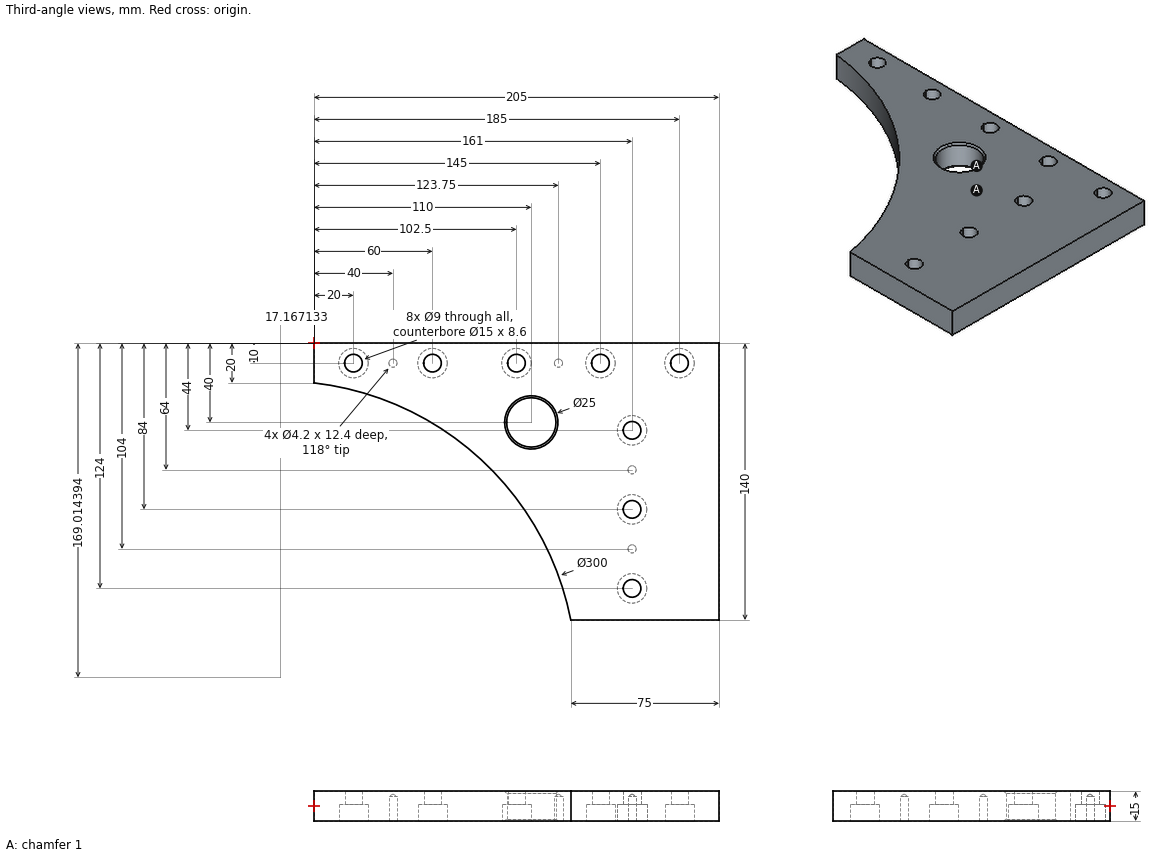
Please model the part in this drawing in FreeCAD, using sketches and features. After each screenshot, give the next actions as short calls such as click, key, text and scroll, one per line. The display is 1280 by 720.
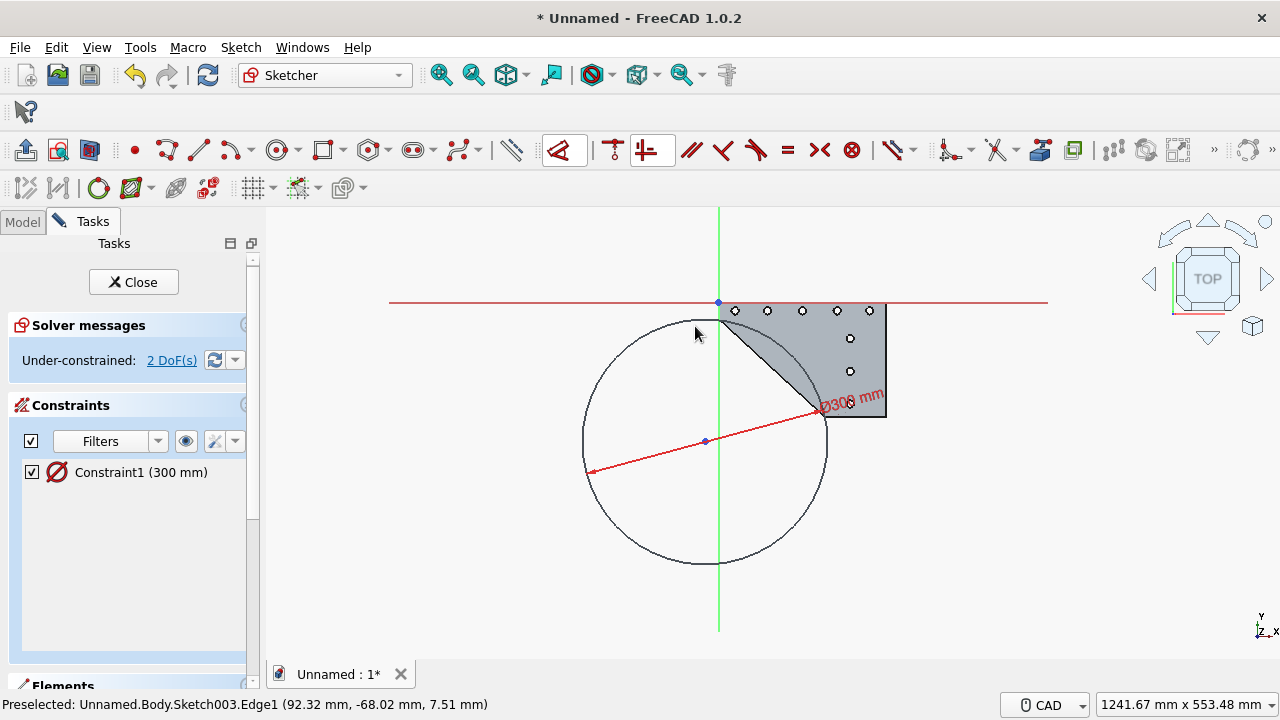
scroll(705, 442, up, 6)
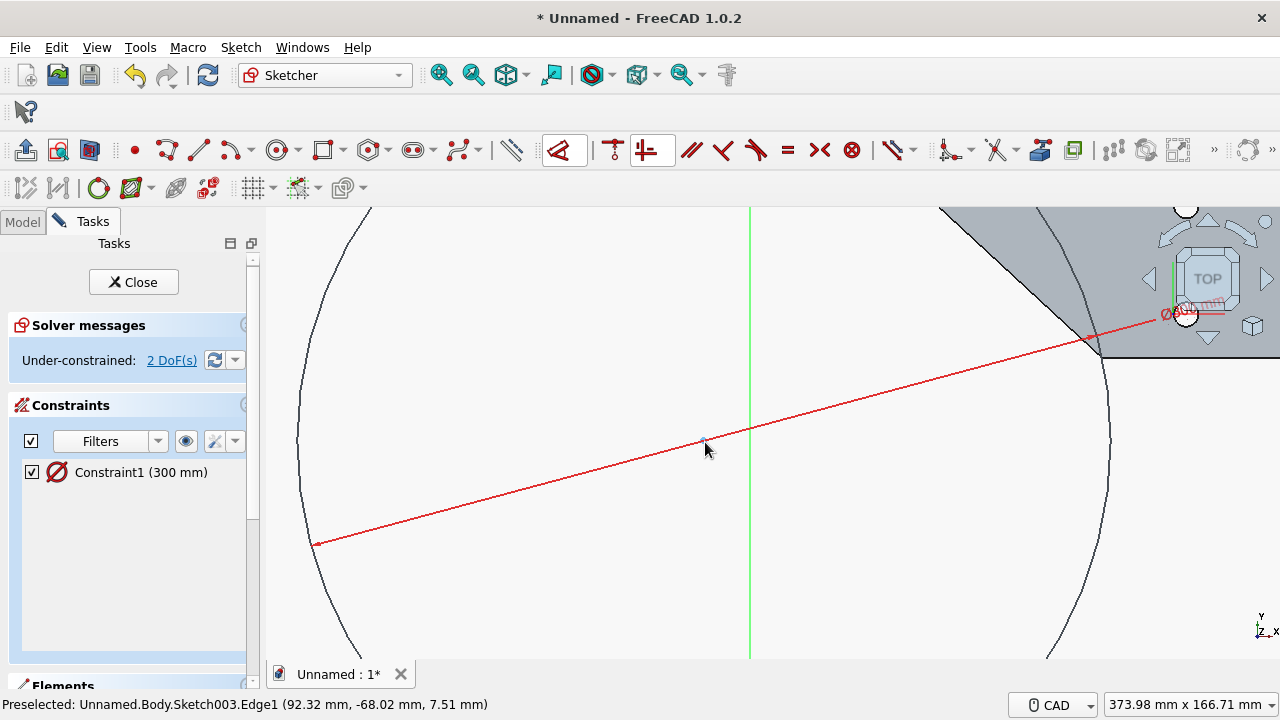
click(704, 441)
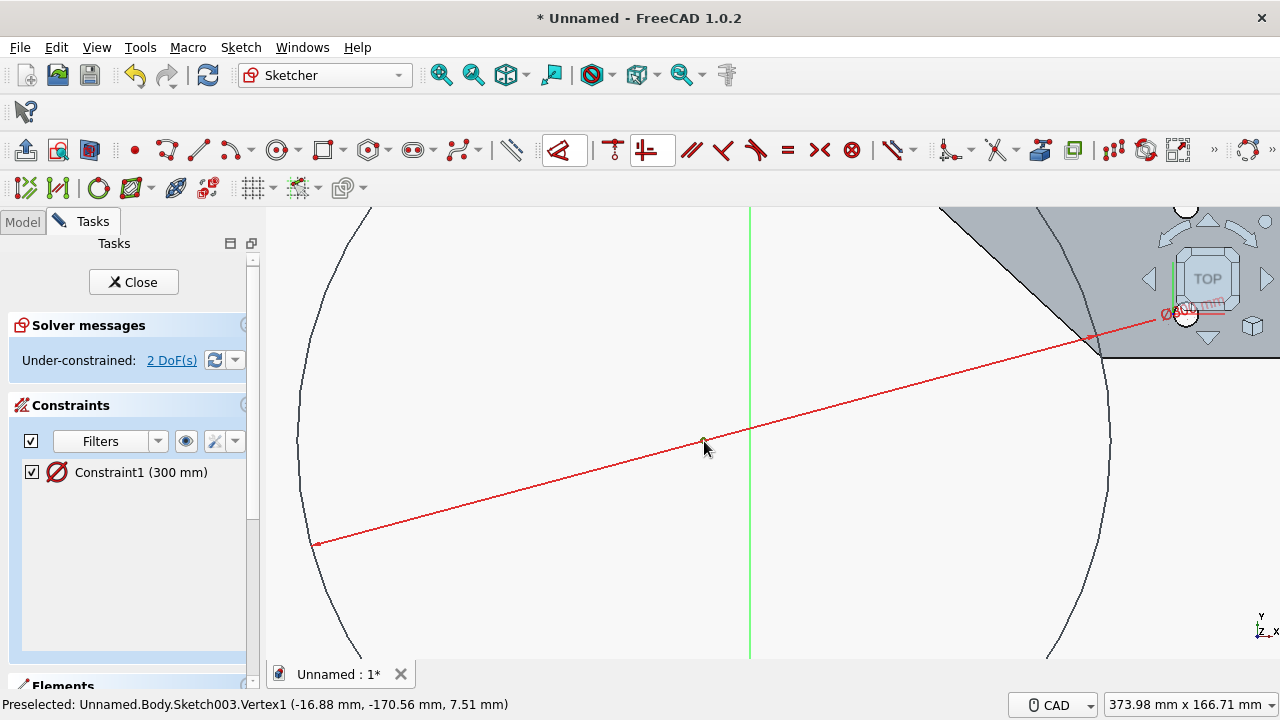
key(l)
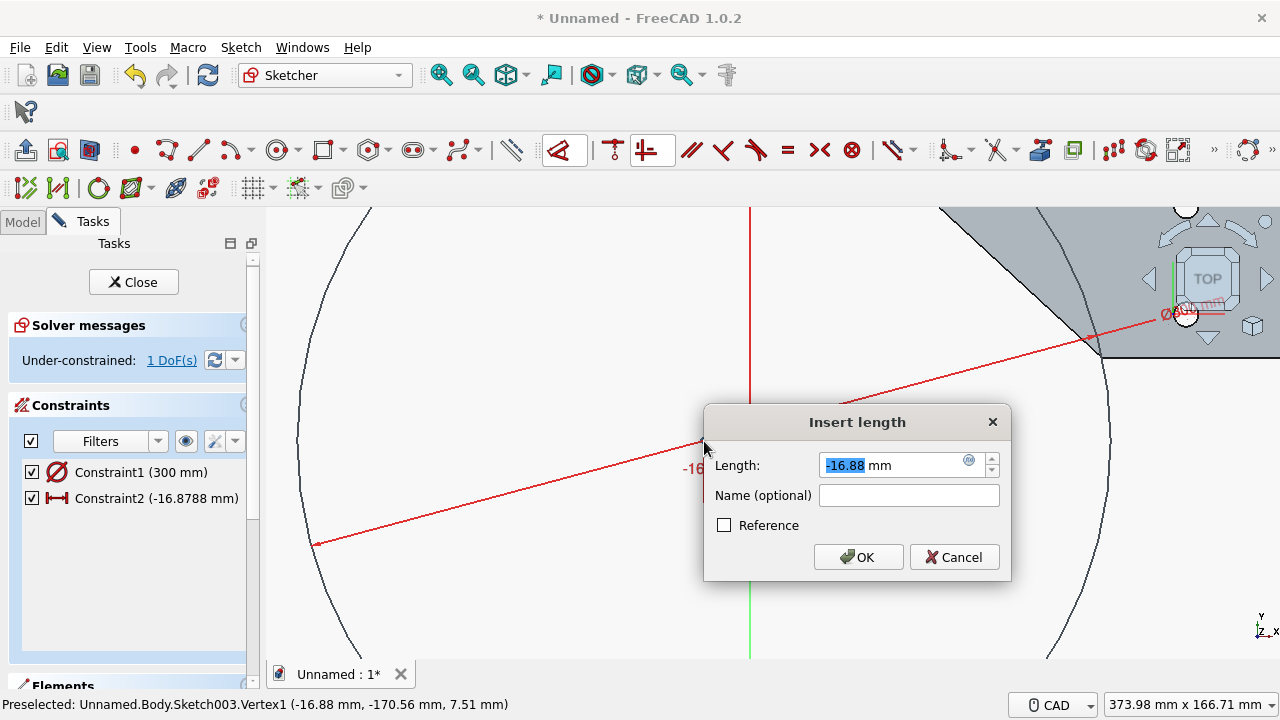
text(-17.167133)
key(Return)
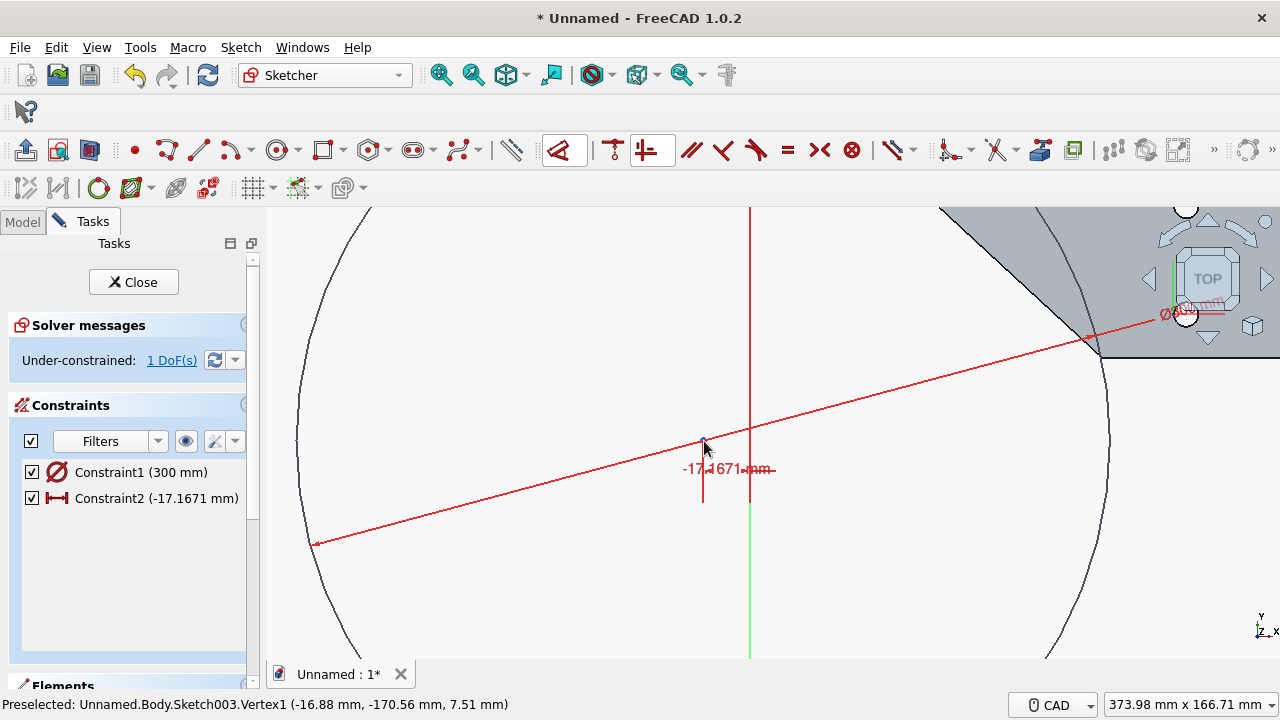
click(703, 441)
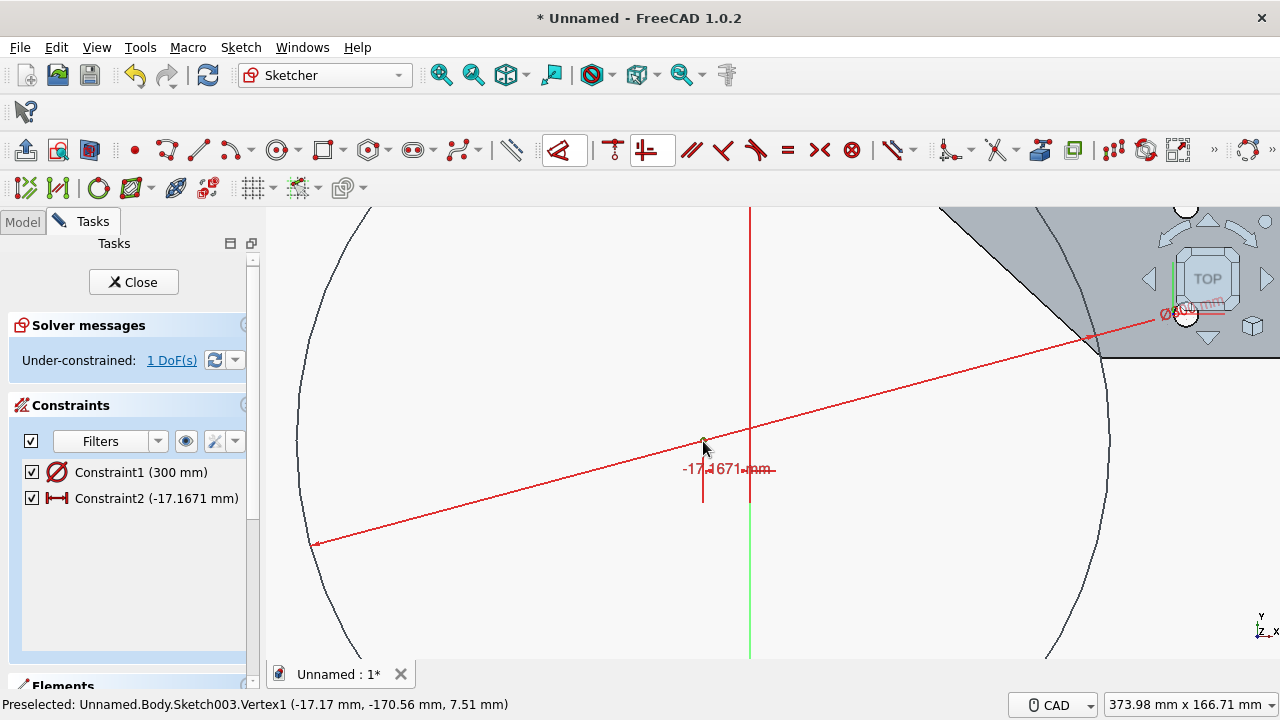
click(582, 150)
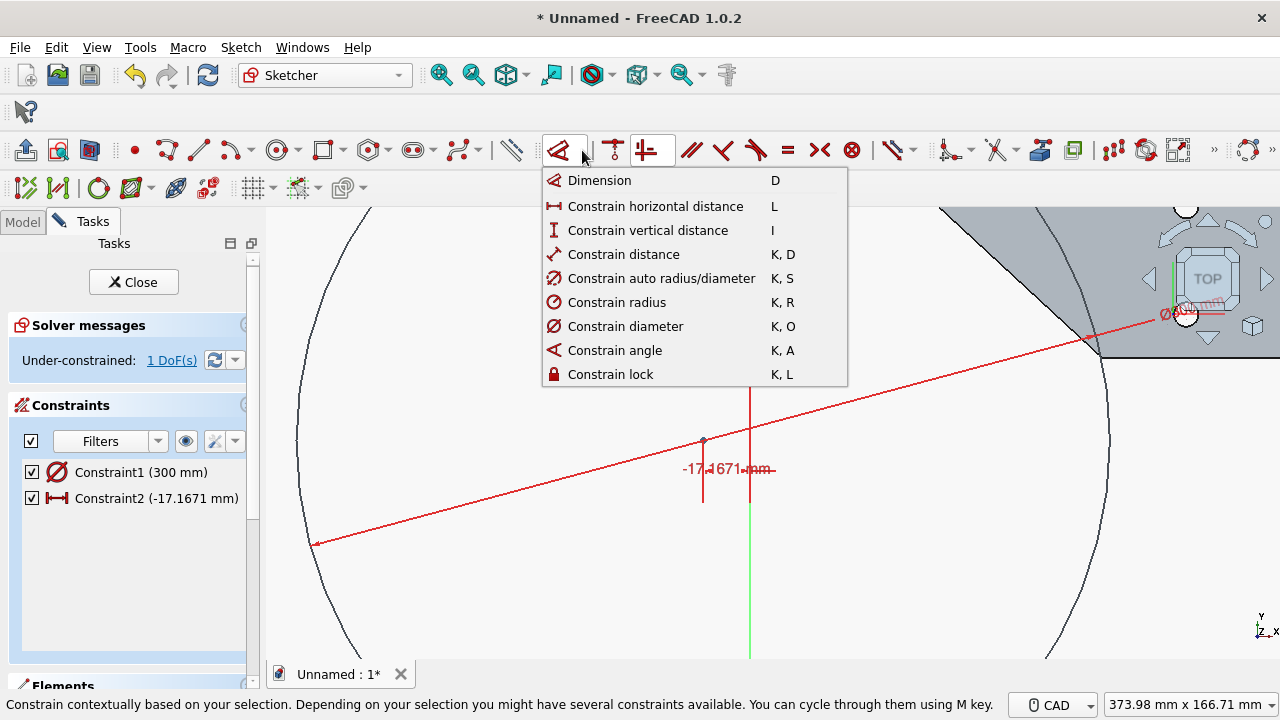
click(695, 230)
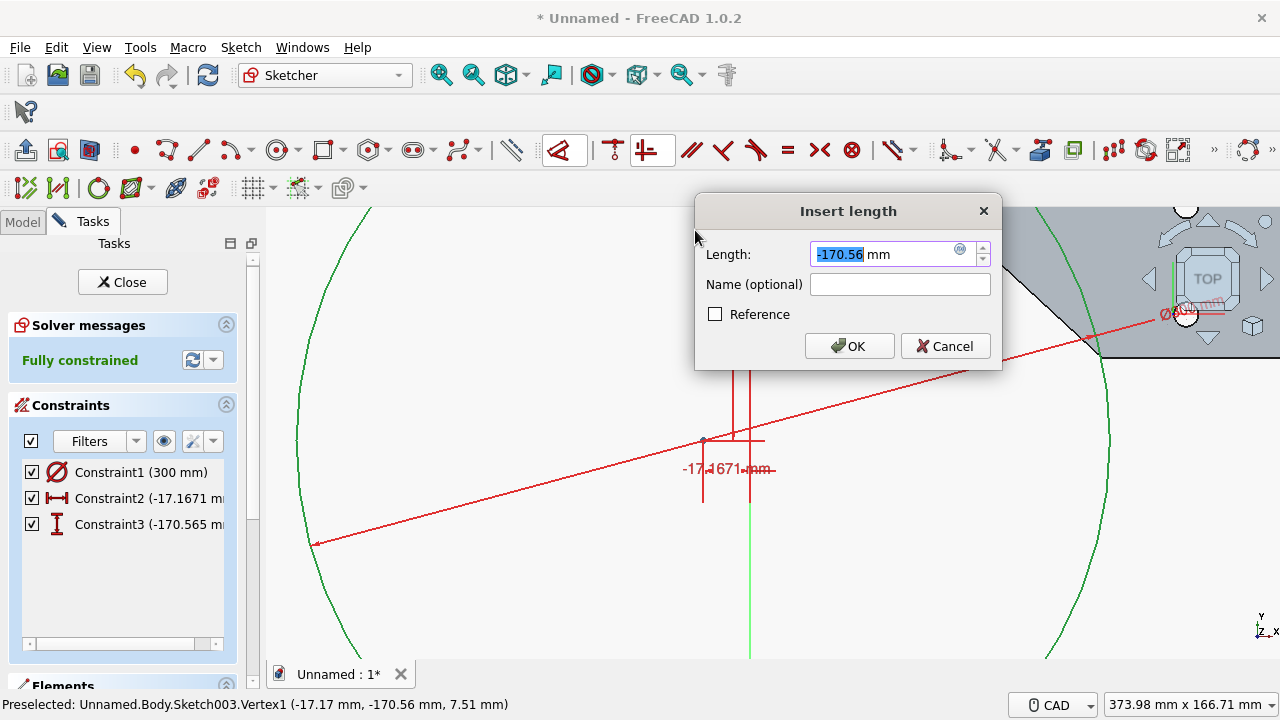
text(-169.014394)
key(Return)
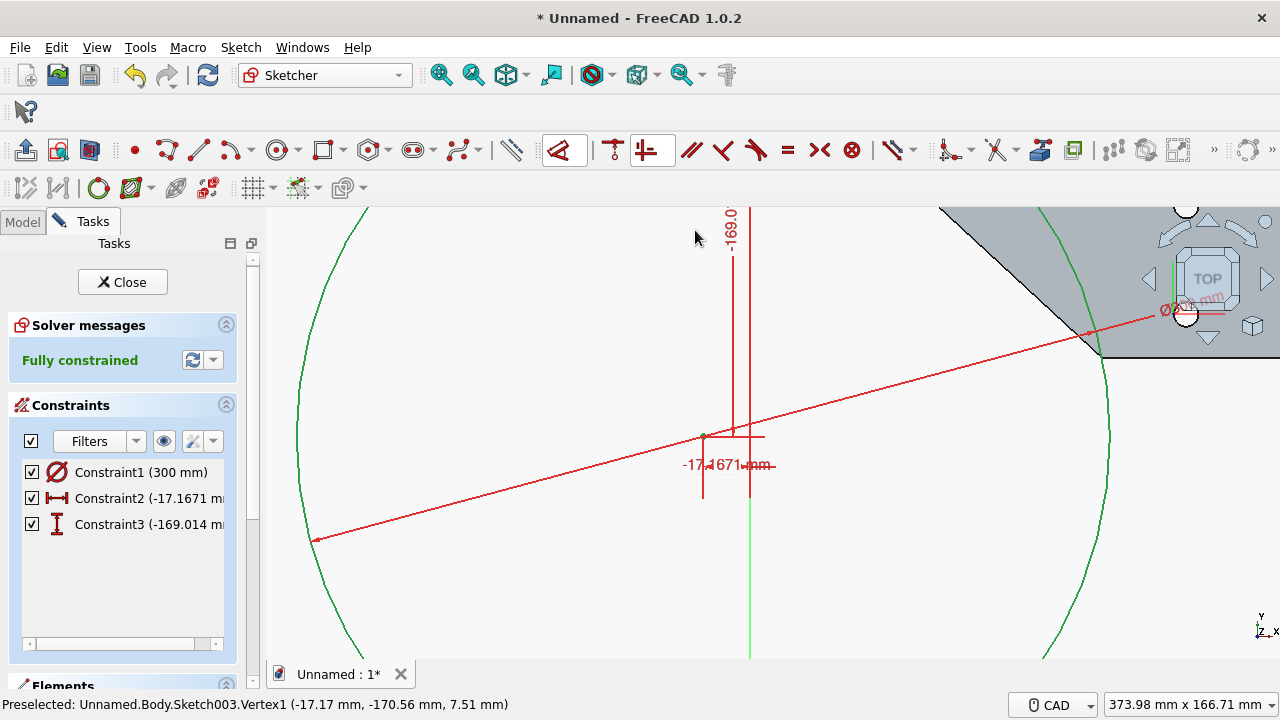
click(123, 282)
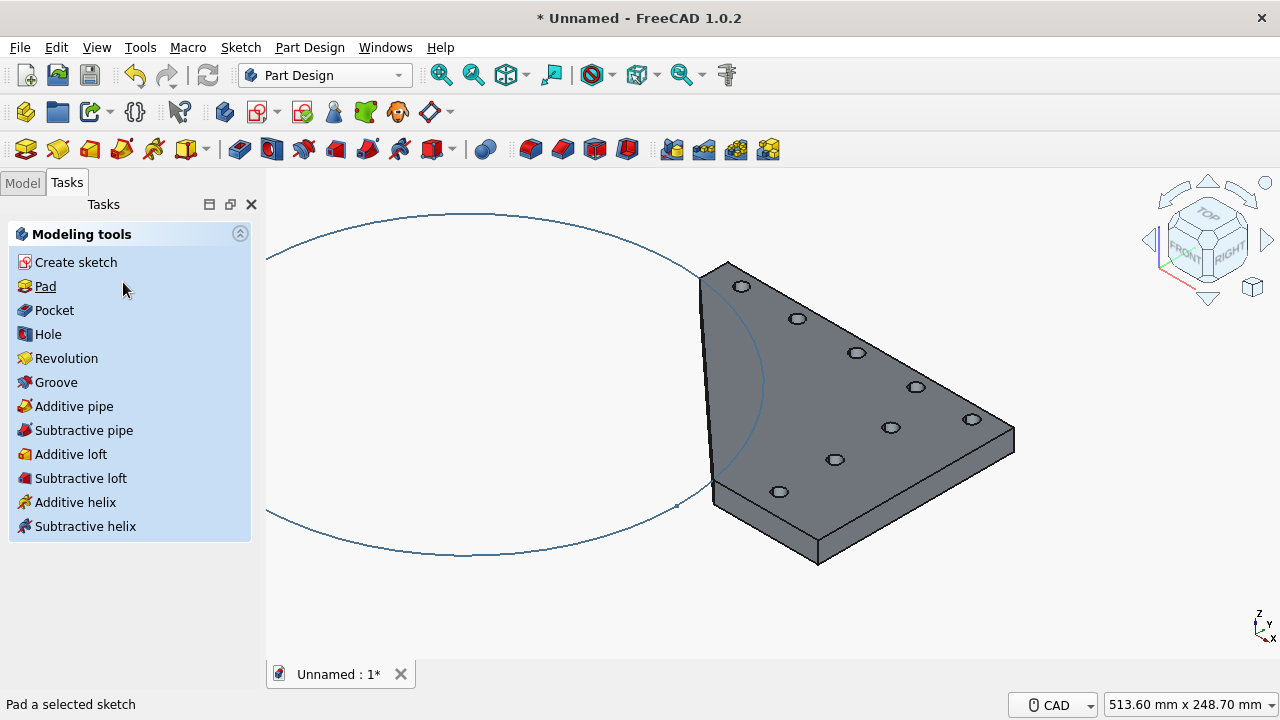
click(240, 150)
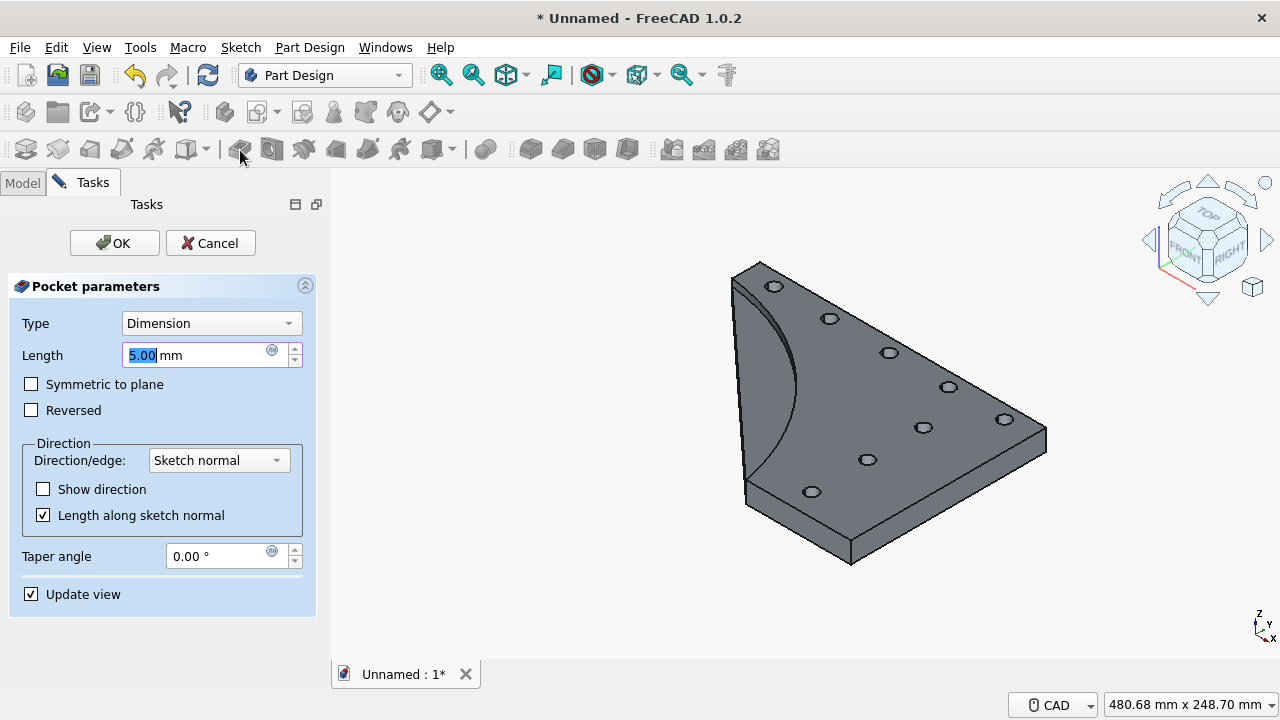
click(212, 324)